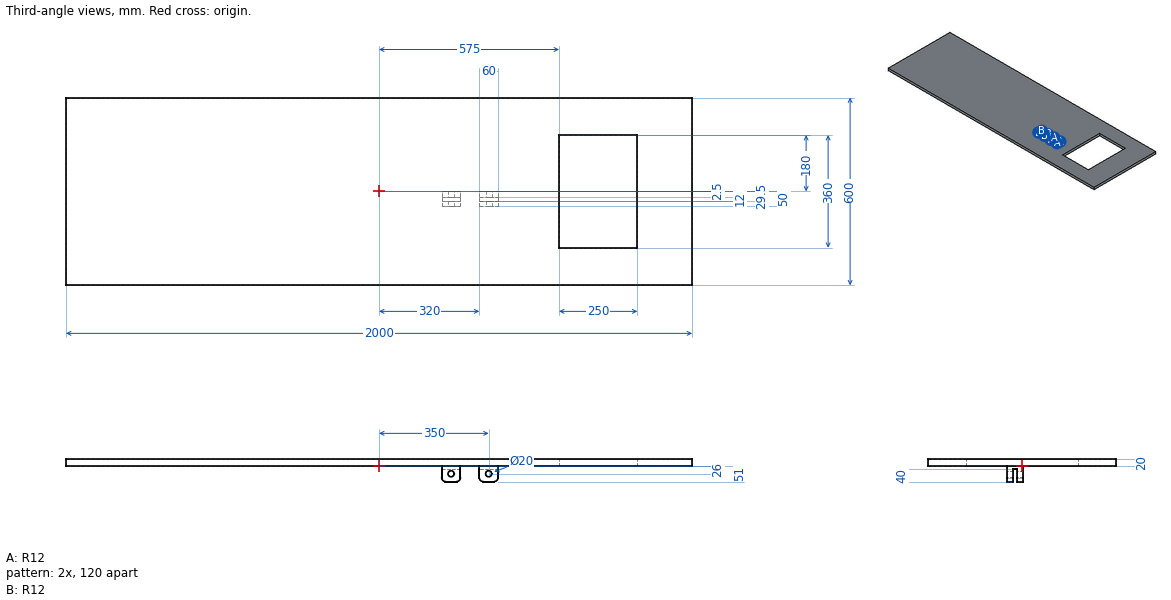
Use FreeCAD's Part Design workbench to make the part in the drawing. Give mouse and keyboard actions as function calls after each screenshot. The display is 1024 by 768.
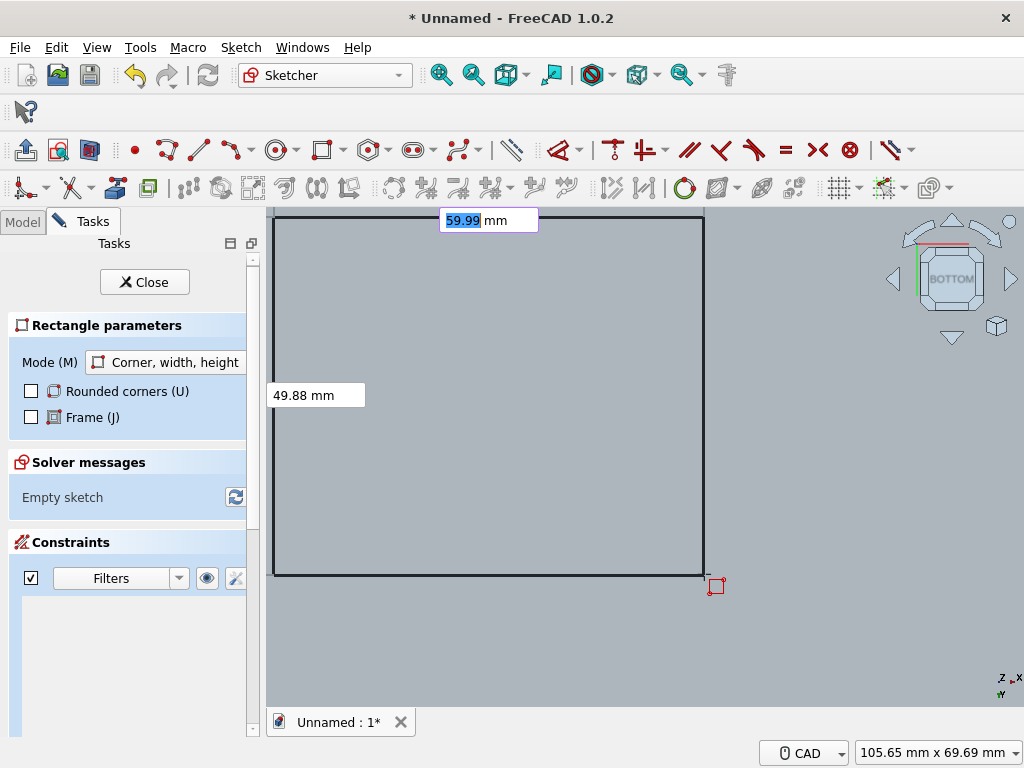
text(60)
key(Tab)
text(50)
key(Return)
key(Escape)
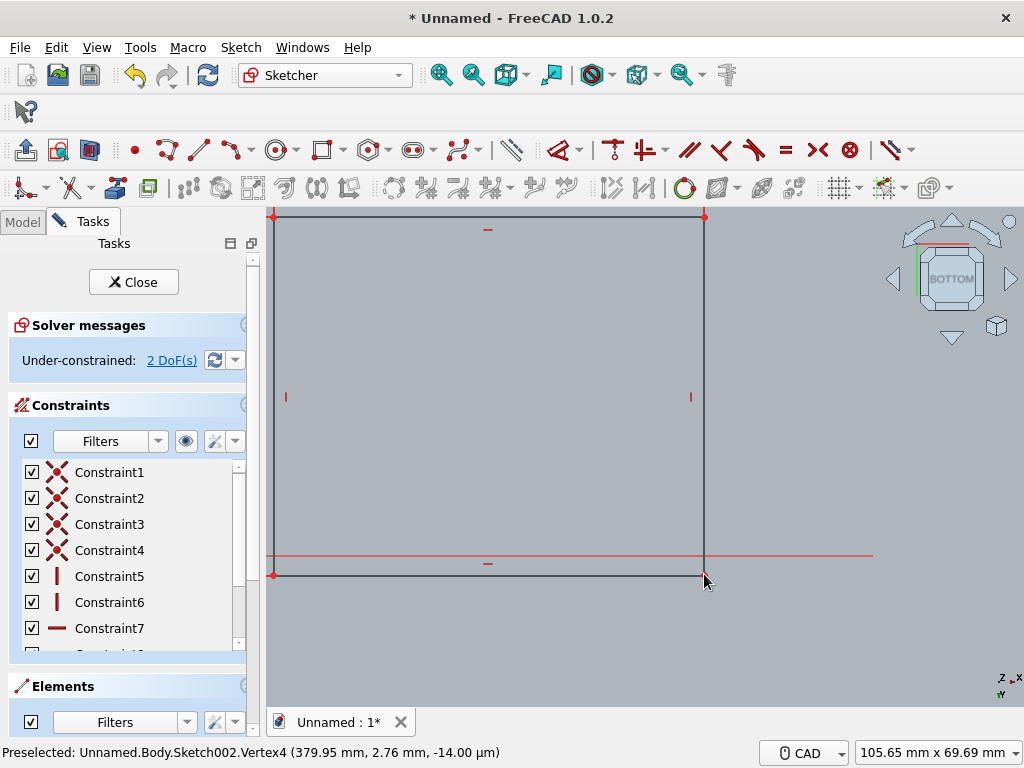
key(d)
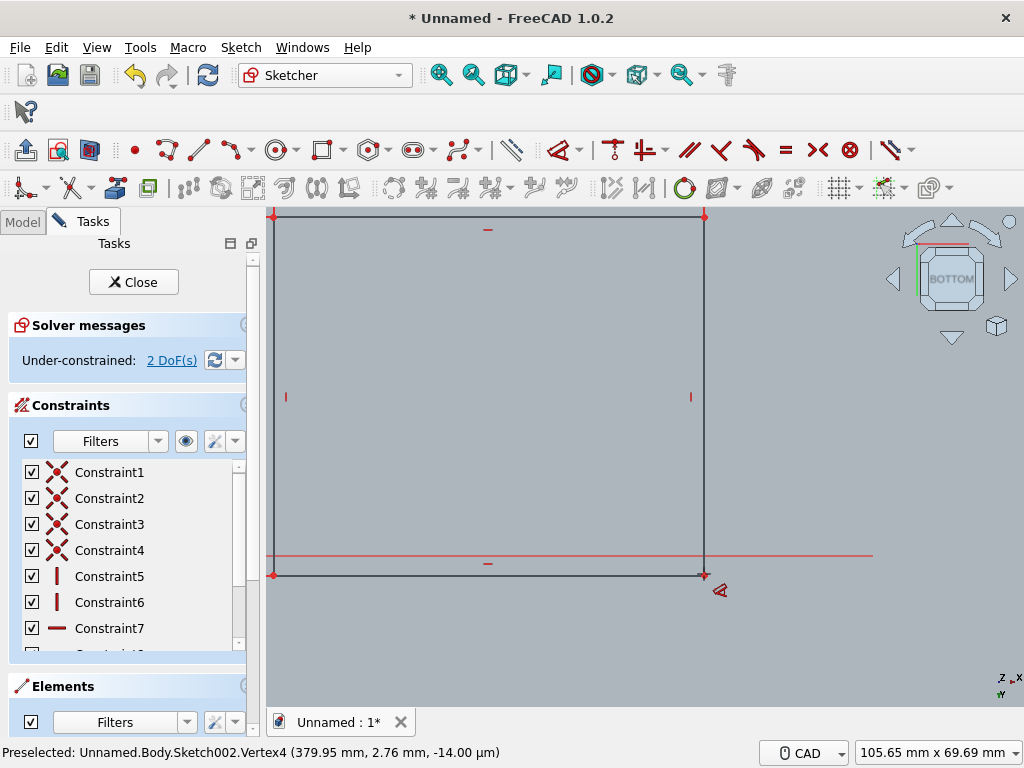
scroll(859, 679, down, 1)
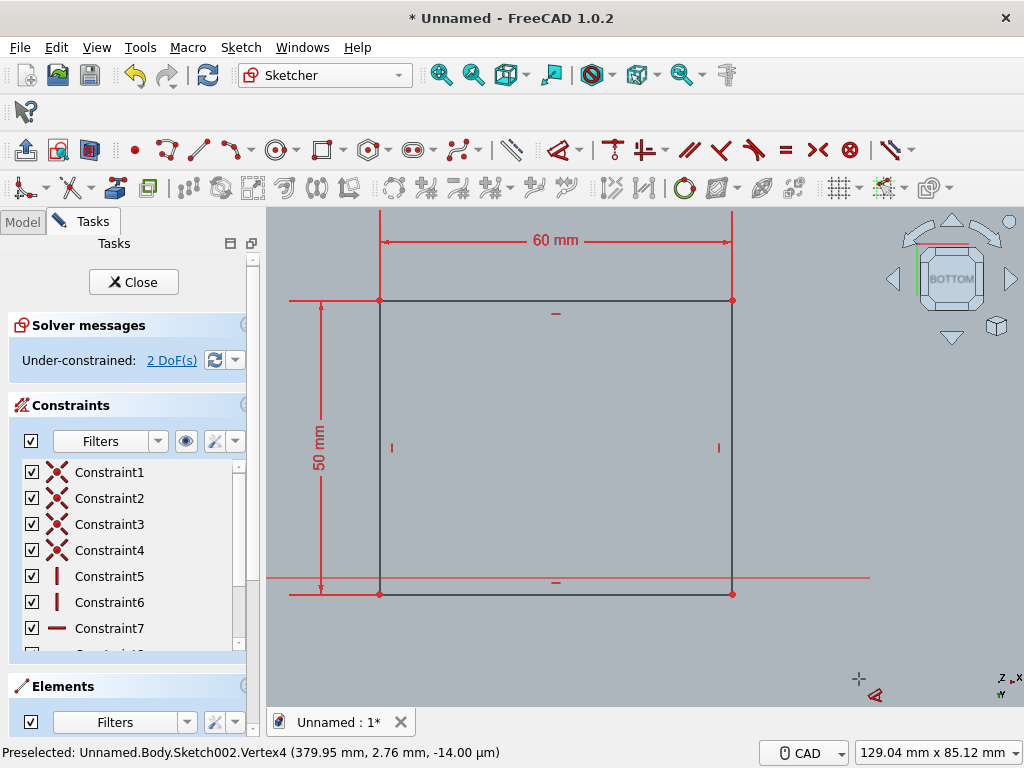
click(380, 301)
click(337, 267)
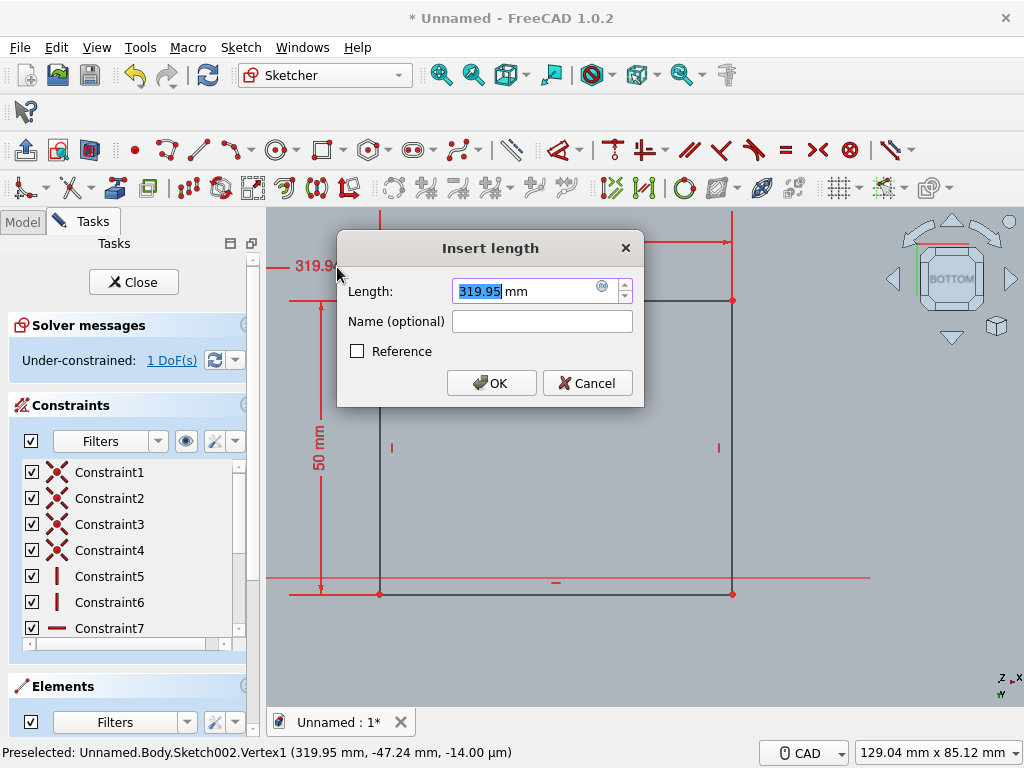
text(320)
key(Return)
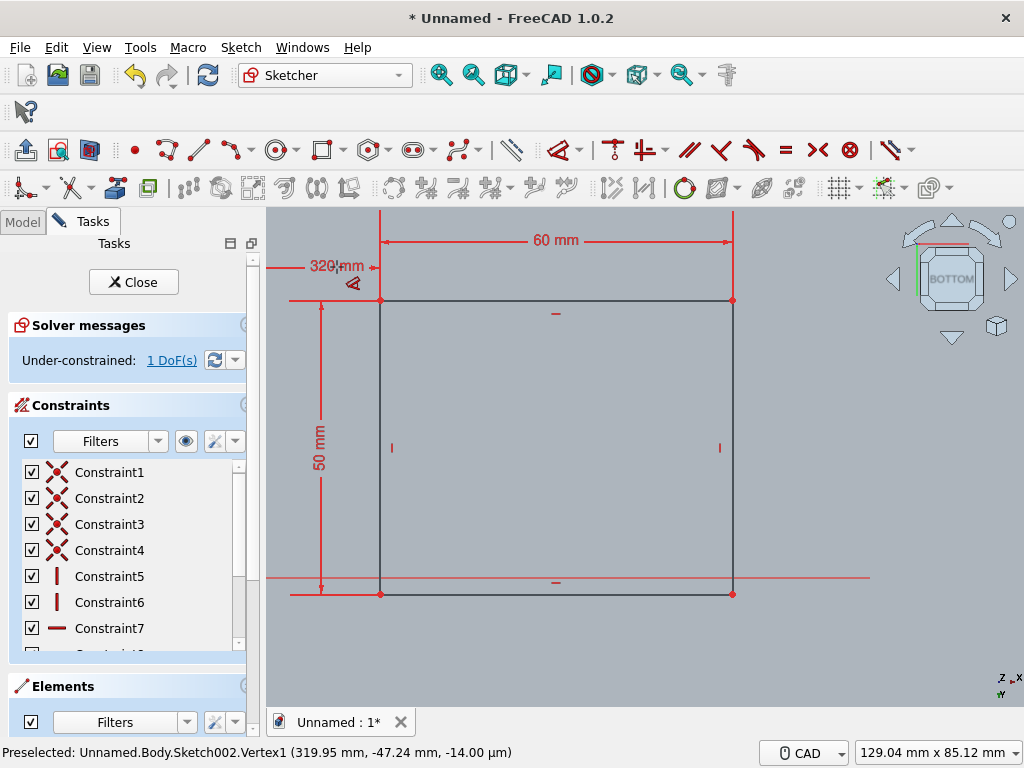
scroll(380, 595, up, 5)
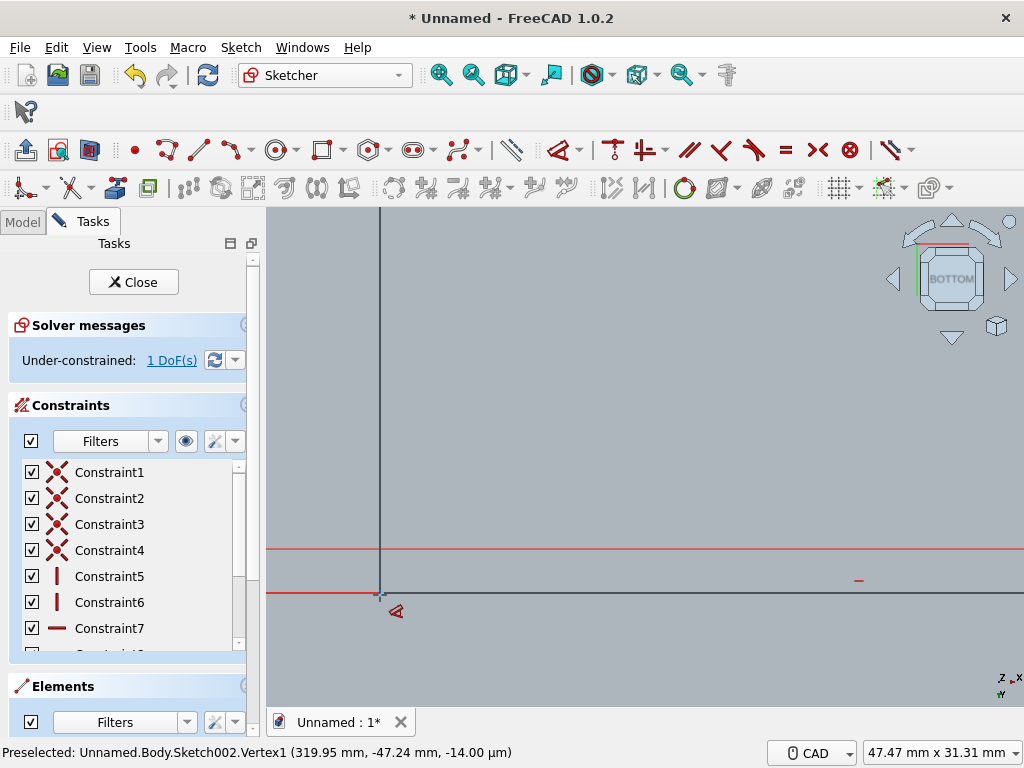
click(380, 593)
click(414, 571)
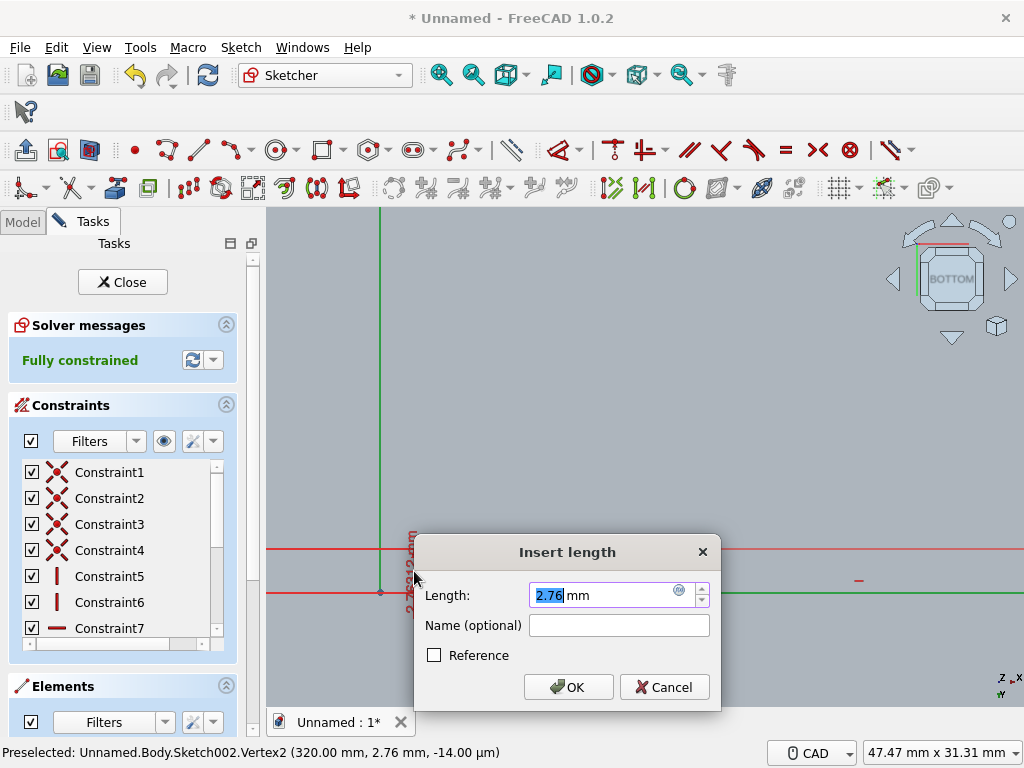
text(2.5)
key(Return)
key(Escape)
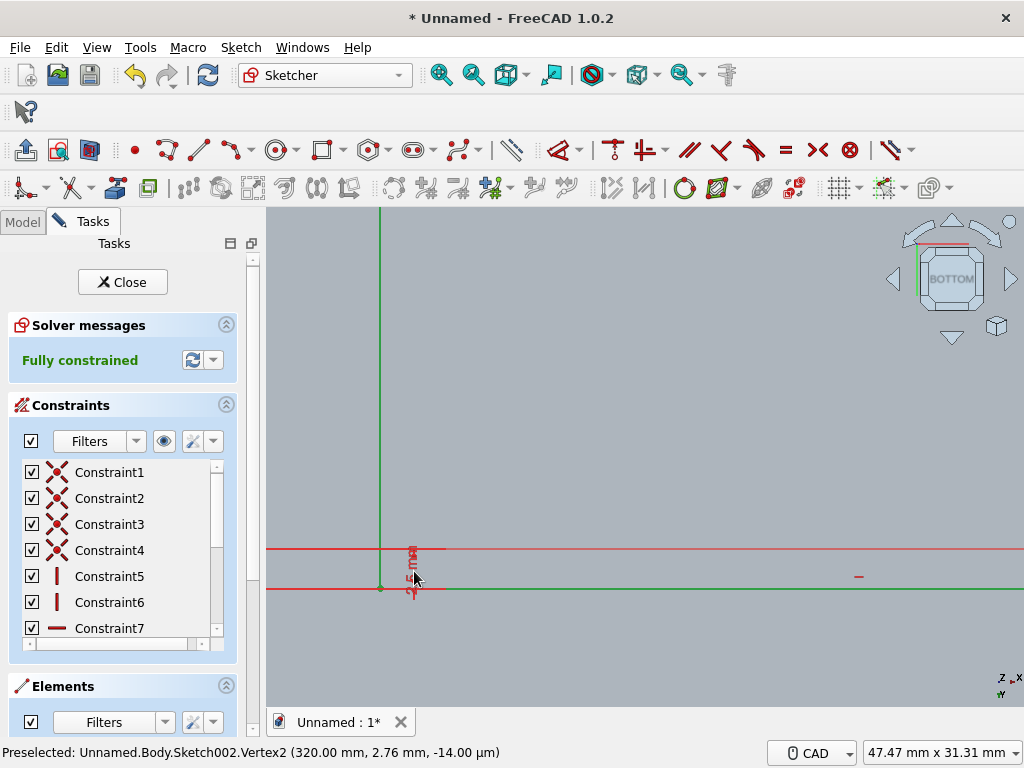
click(123, 282)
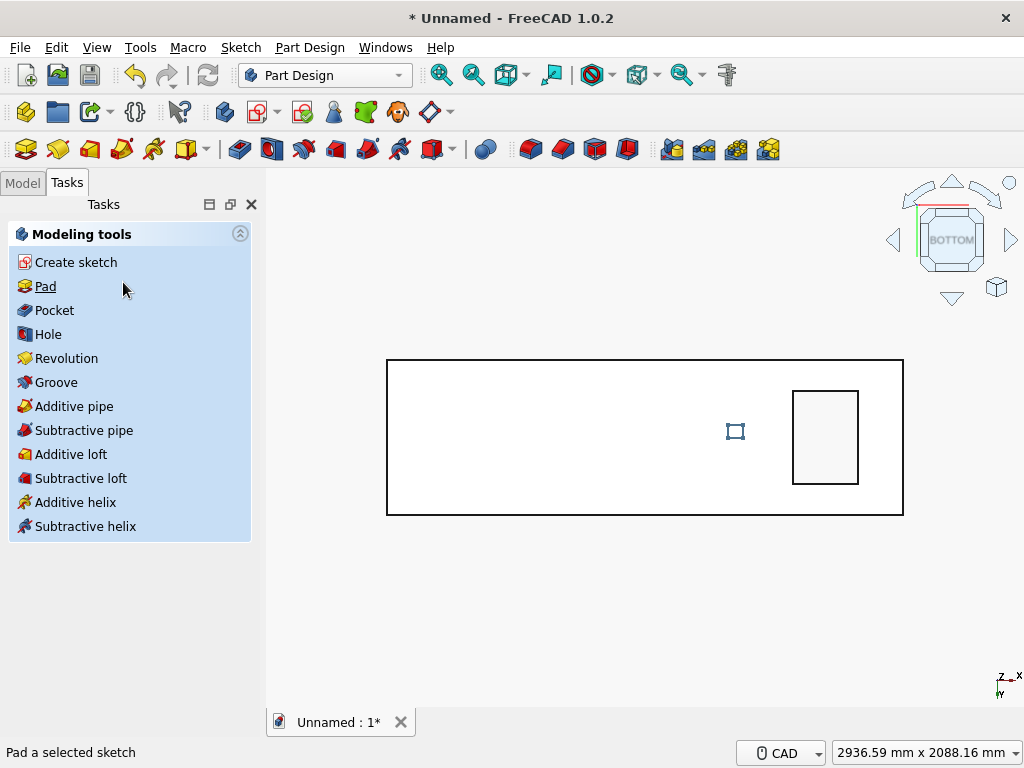
click(26, 150)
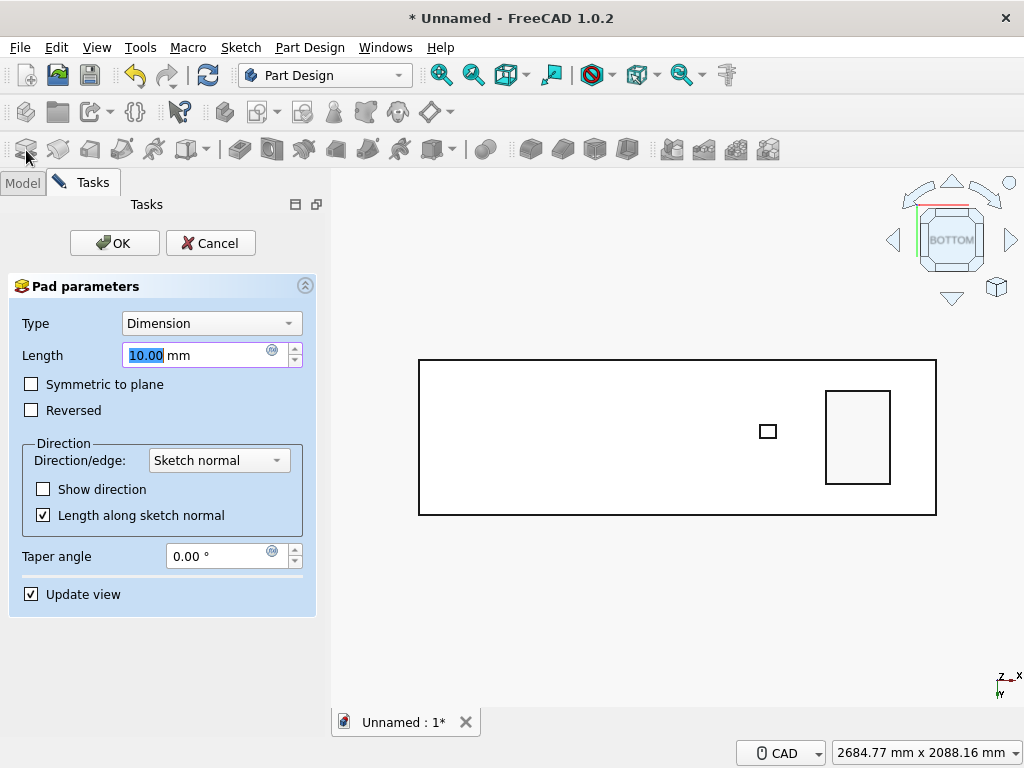
text(51)
key(Tab)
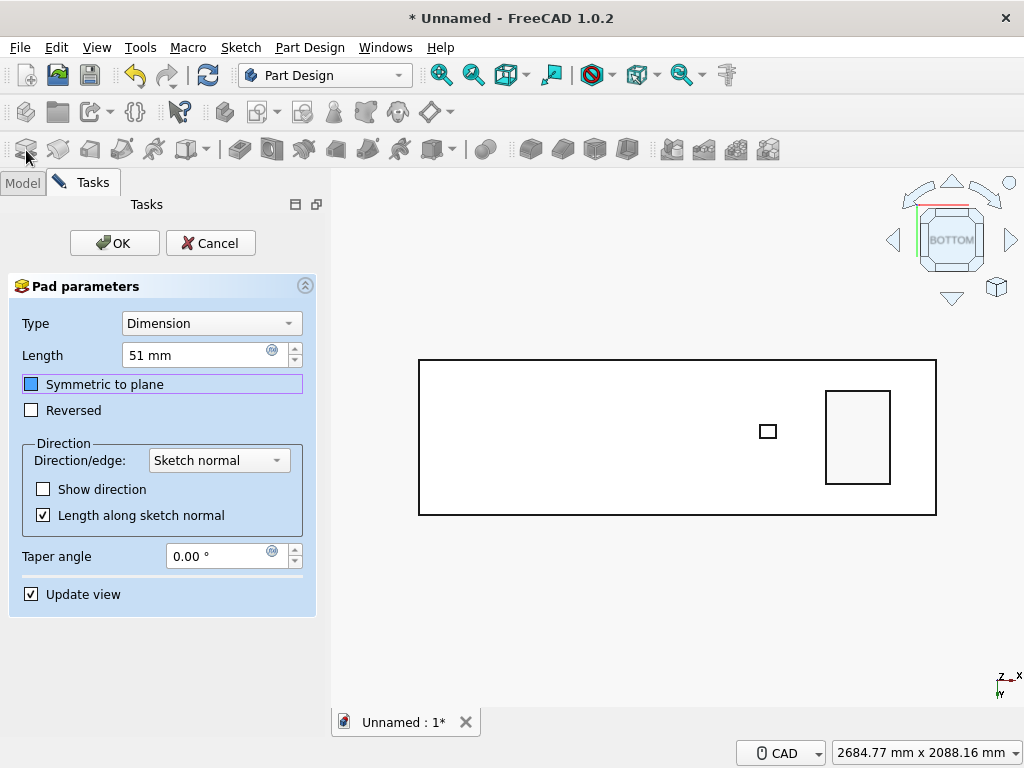
click(115, 243)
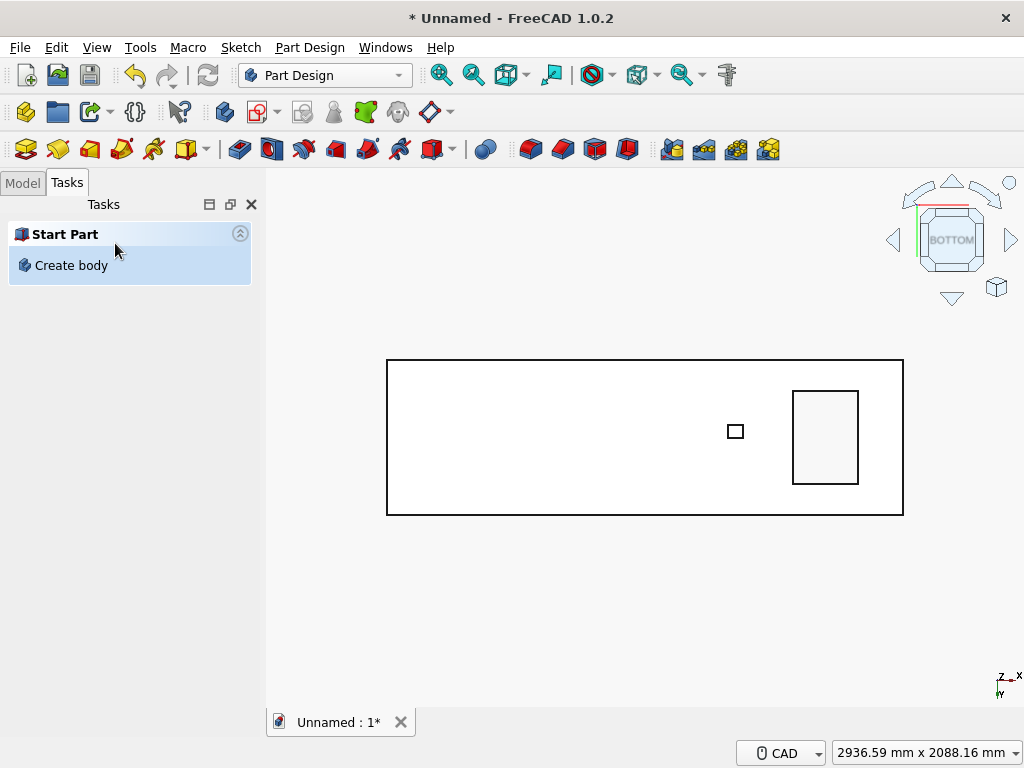
scroll(735, 431, up, 4)